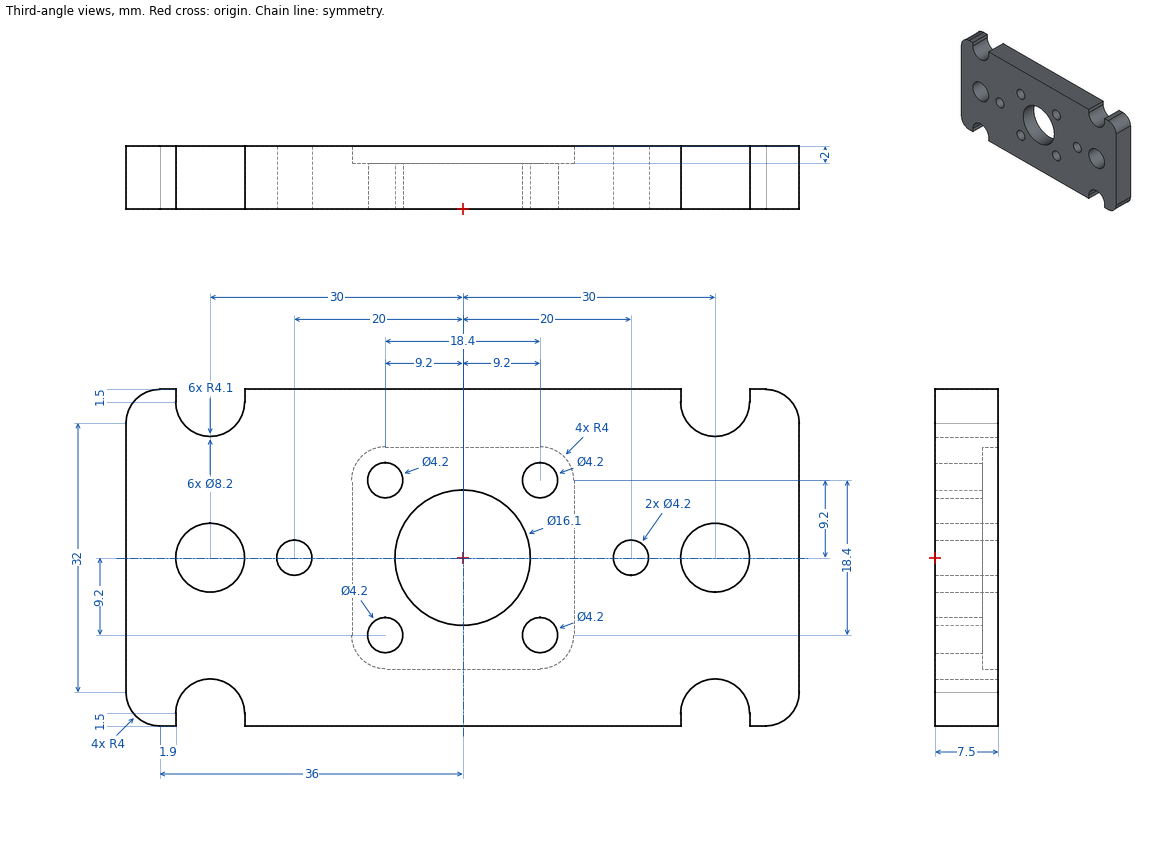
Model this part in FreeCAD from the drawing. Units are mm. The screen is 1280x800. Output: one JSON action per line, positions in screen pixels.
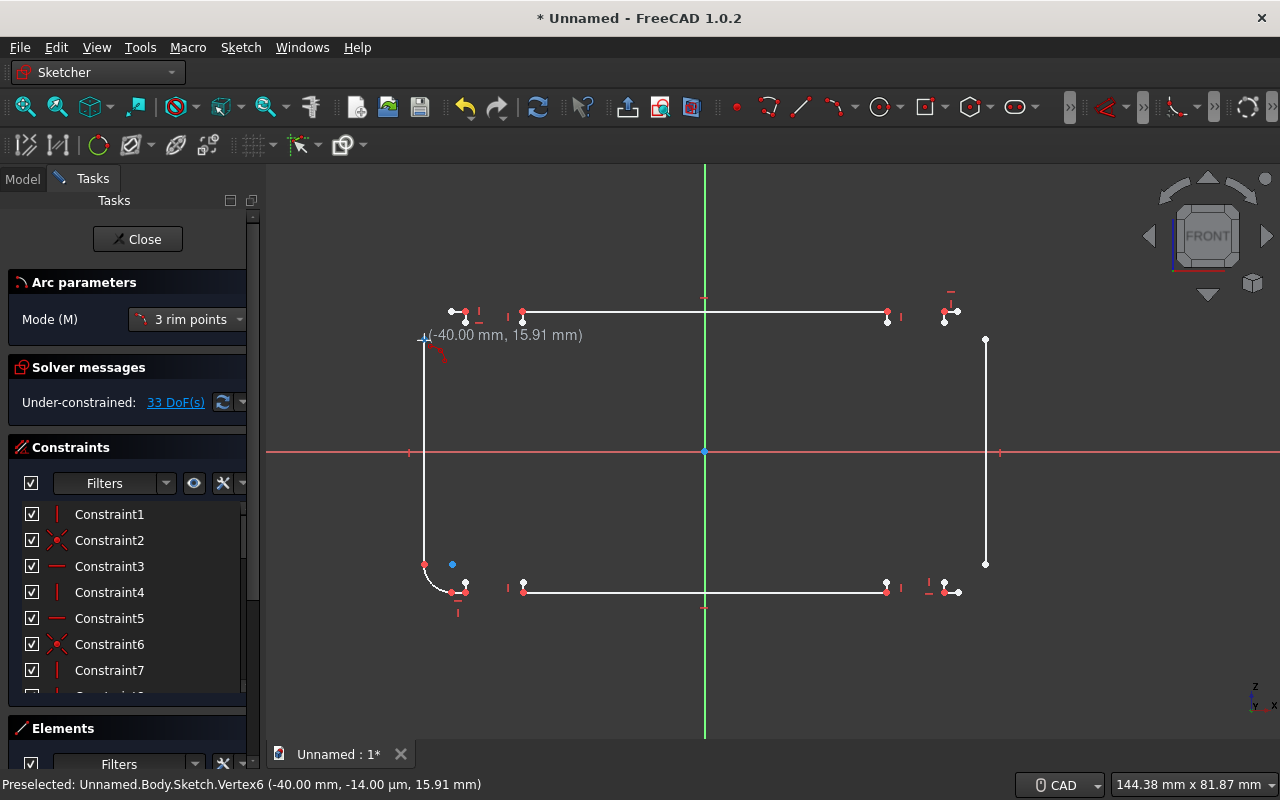
{"action": "scroll", "coordinate": [452, 311], "scroll_direction": "up", "scroll_amount": 5}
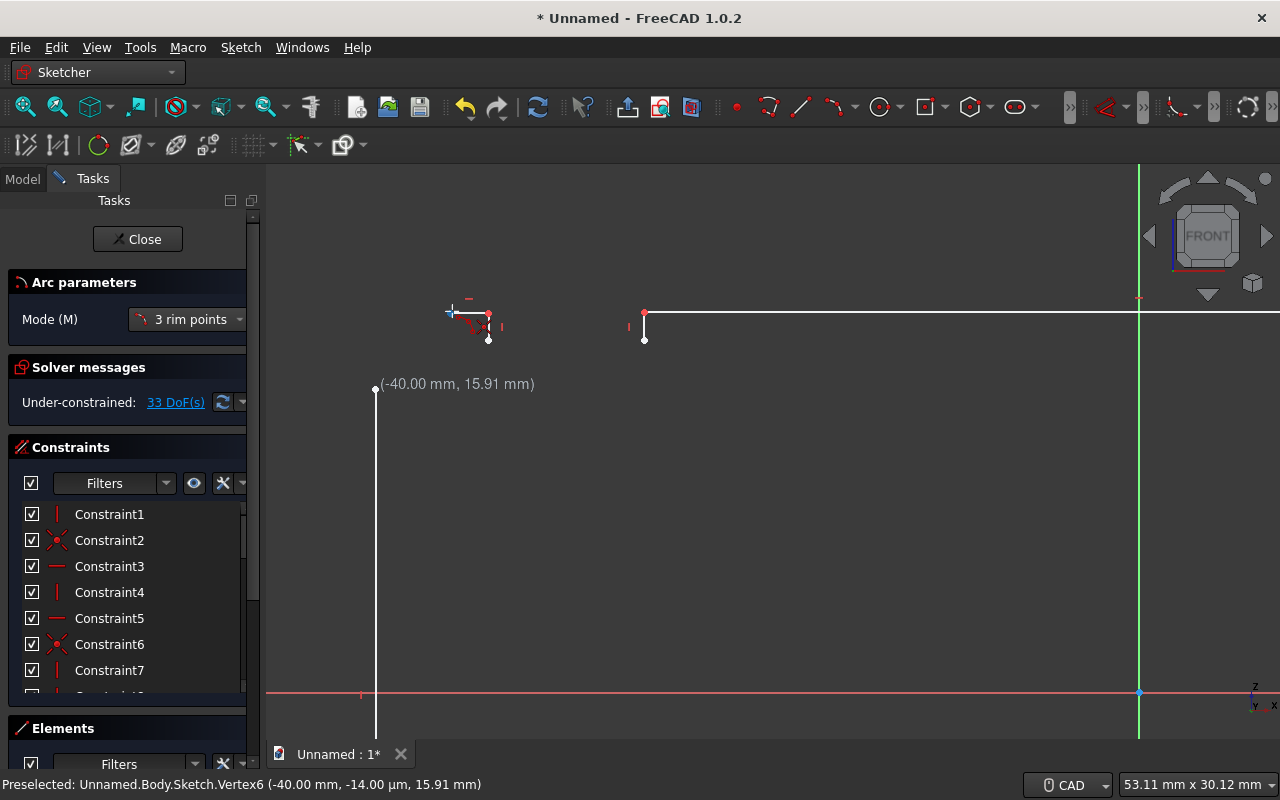
{"action": "left_click", "coordinate": [451, 313]}
{"action": "left_click", "coordinate": [398, 333]}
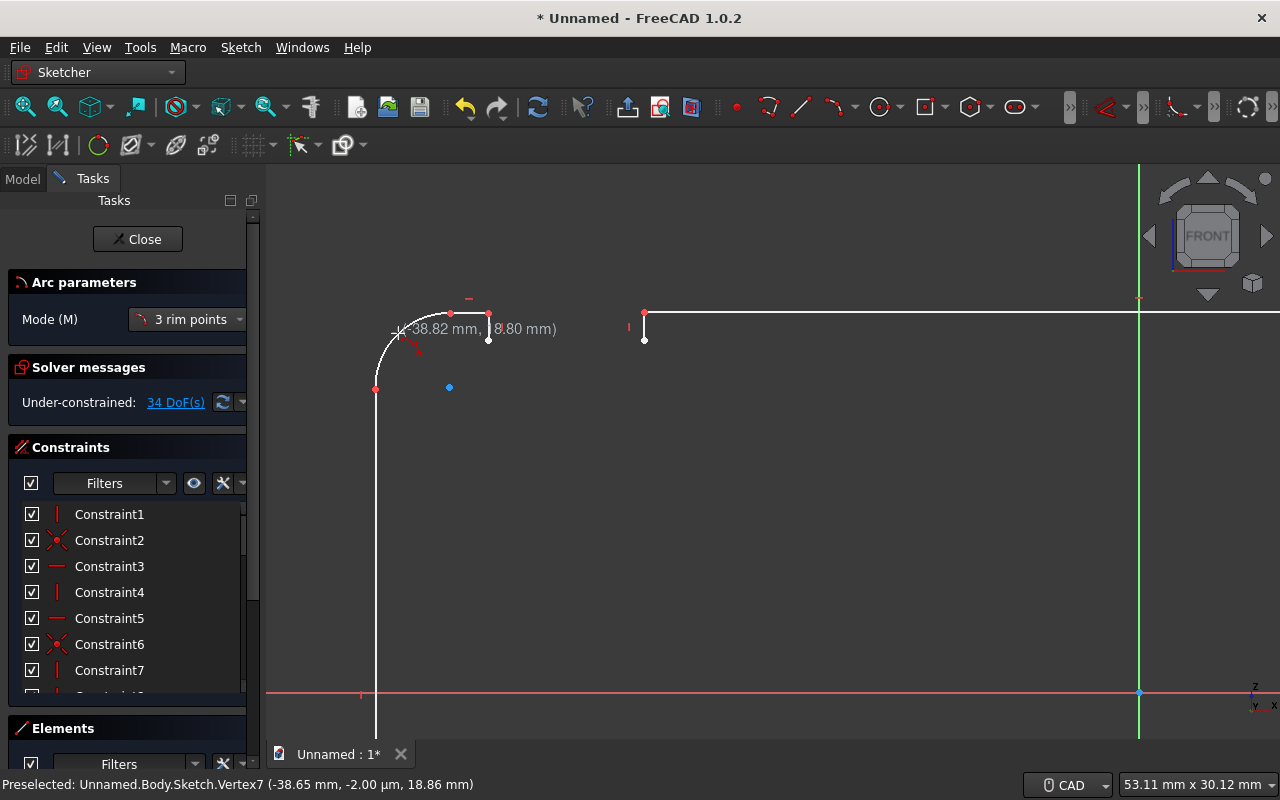
{"action": "left_click", "coordinate": [489, 341]}
{"action": "left_click", "coordinate": [644, 341]}
{"action": "left_click", "coordinate": [566, 418]}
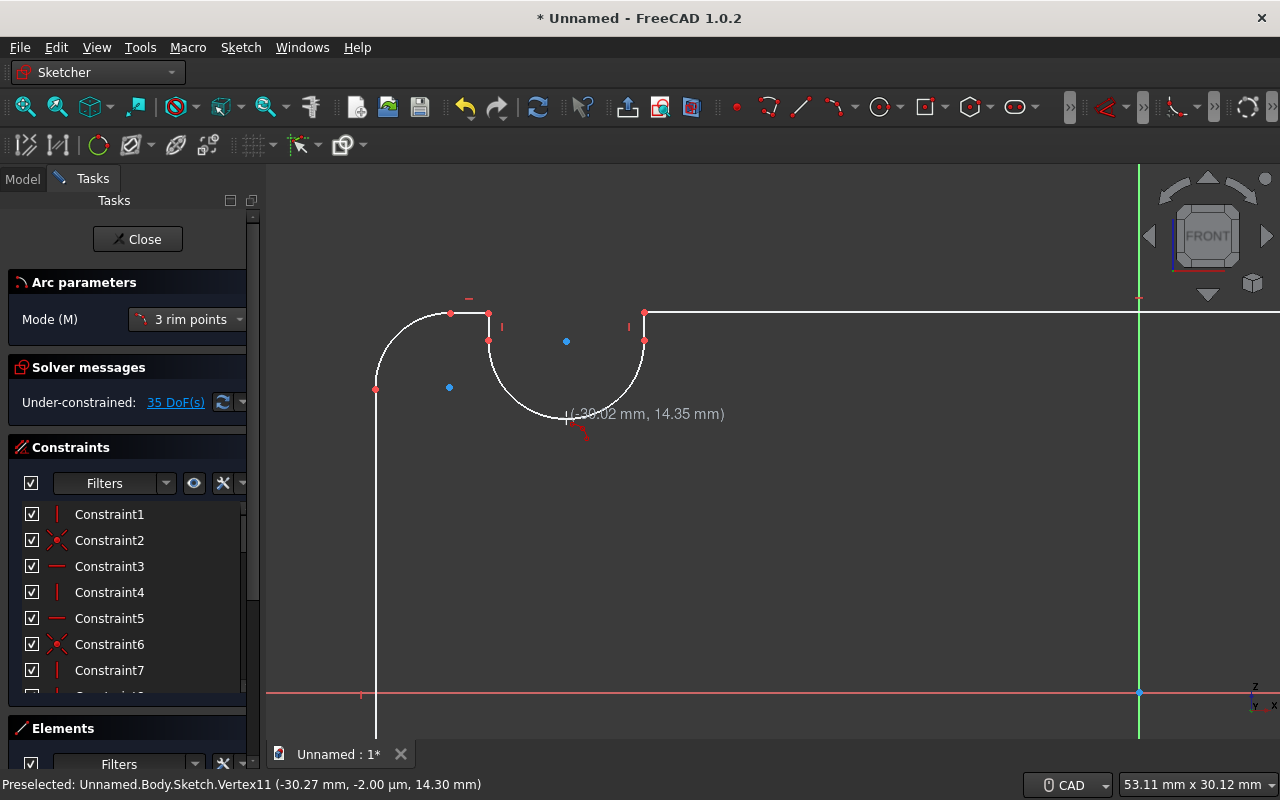
{"action": "scroll", "coordinate": [452, 311], "scroll_direction": "down", "scroll_amount": 5}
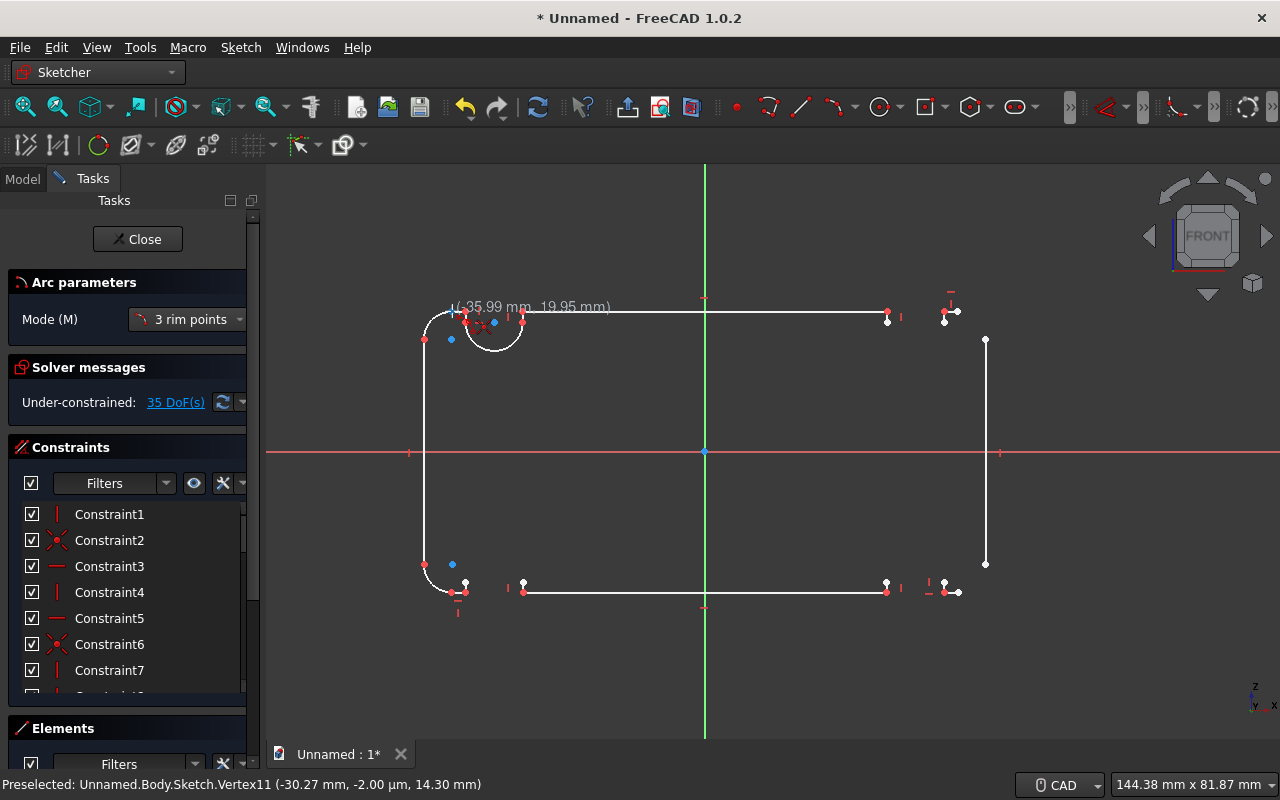
{"action": "scroll", "coordinate": [887, 322], "scroll_direction": "up", "scroll_amount": 6}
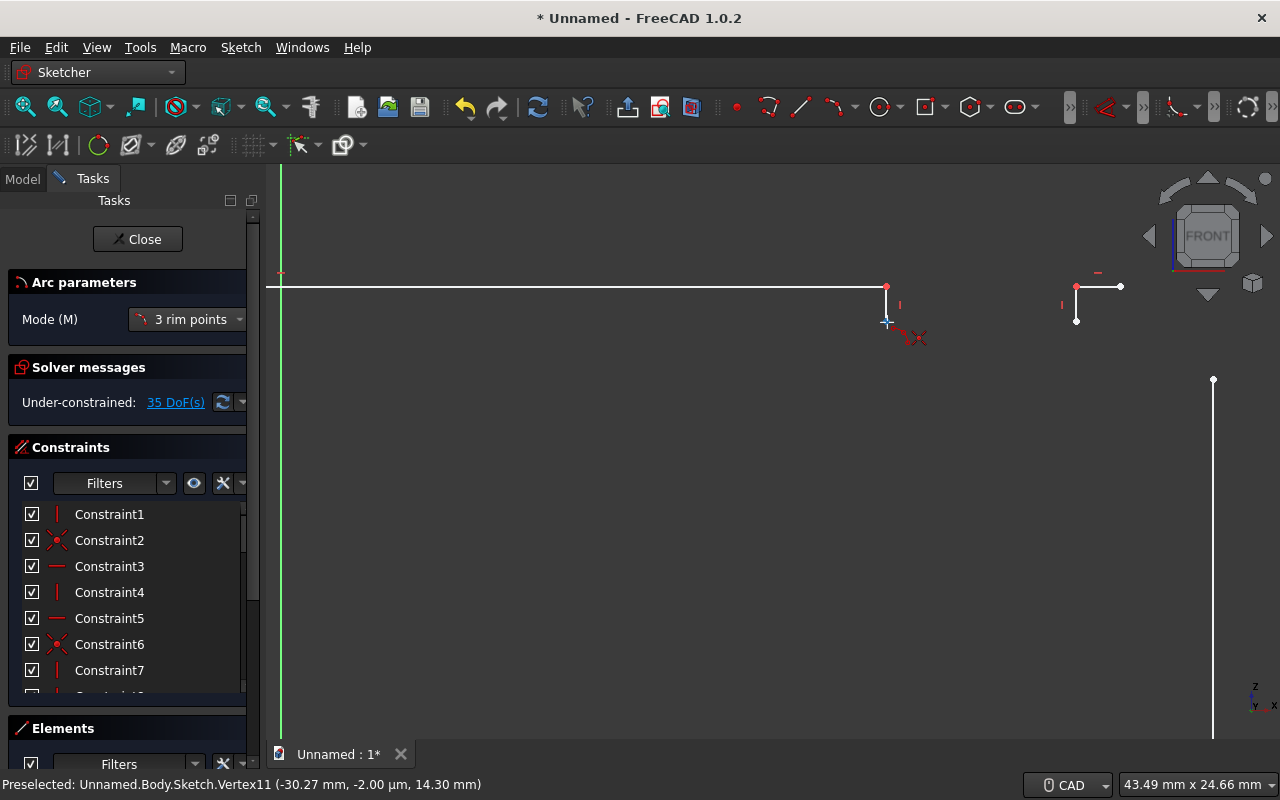
{"action": "left_click", "coordinate": [886, 321]}
{"action": "left_click", "coordinate": [1076, 321]}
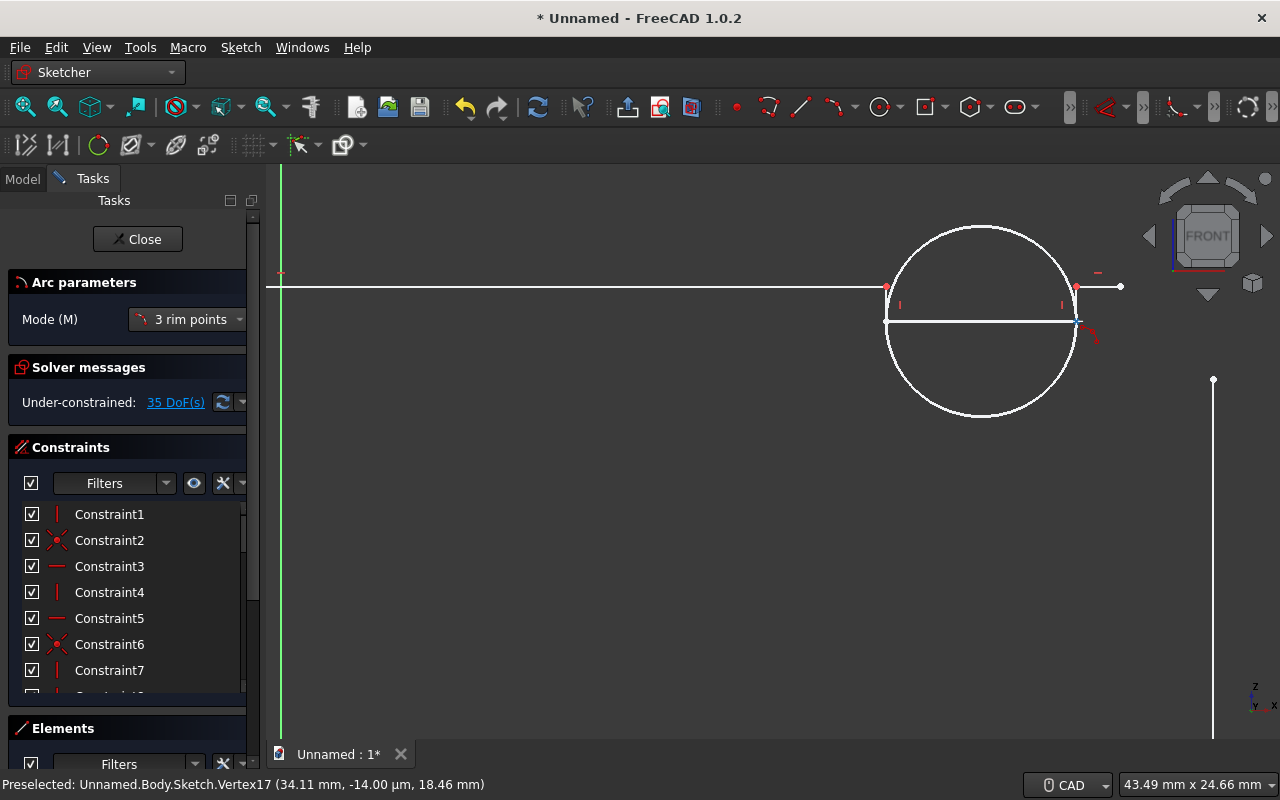
{"action": "scroll", "coordinate": [887, 322], "scroll_direction": "down", "scroll_amount": 6}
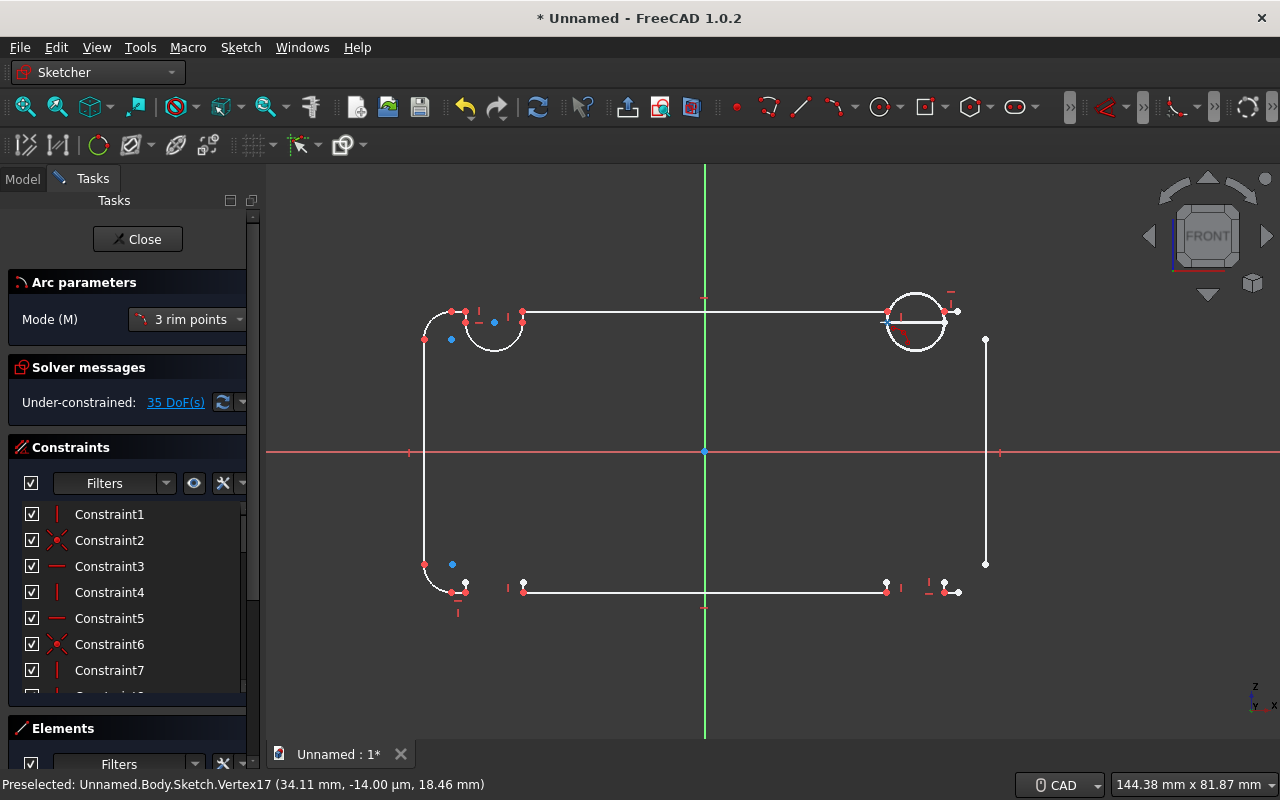
{"action": "left_click", "coordinate": [916, 351]}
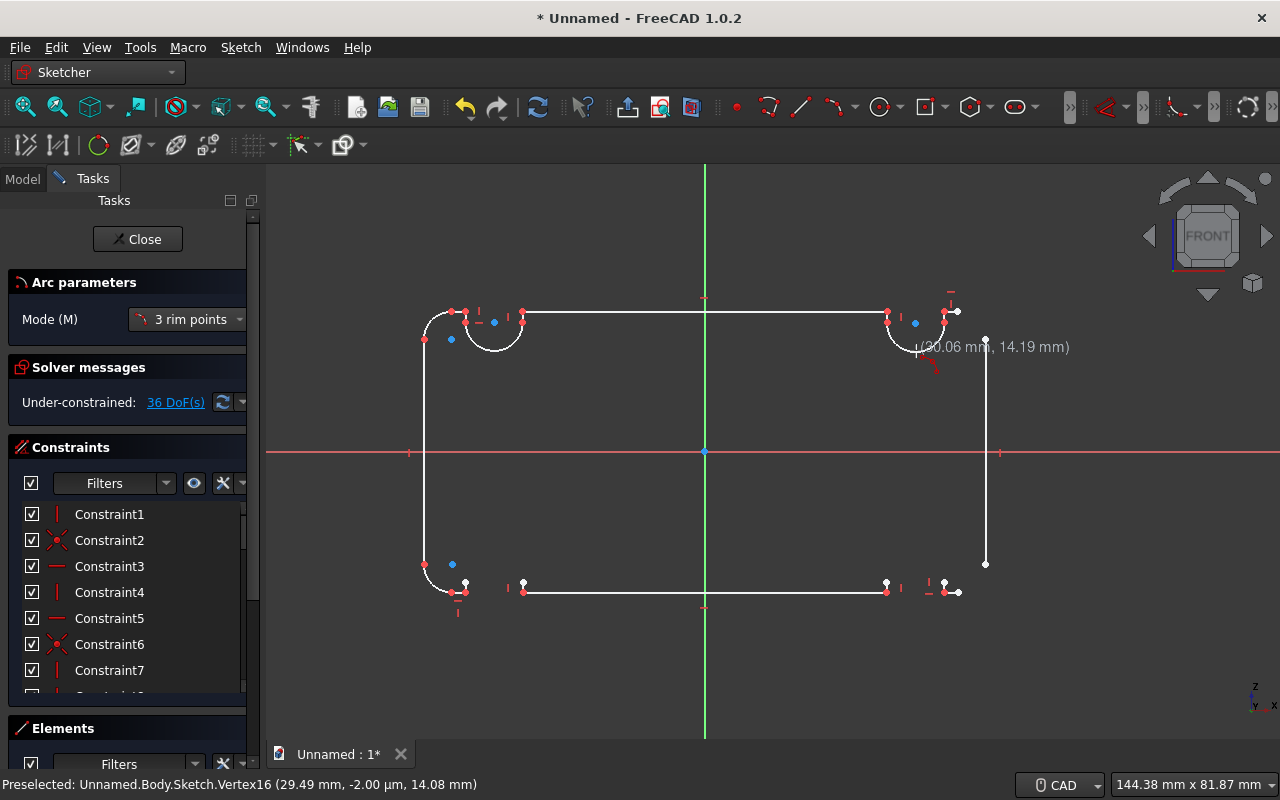
{"action": "scroll", "coordinate": [958, 311], "scroll_direction": "up", "scroll_amount": 5}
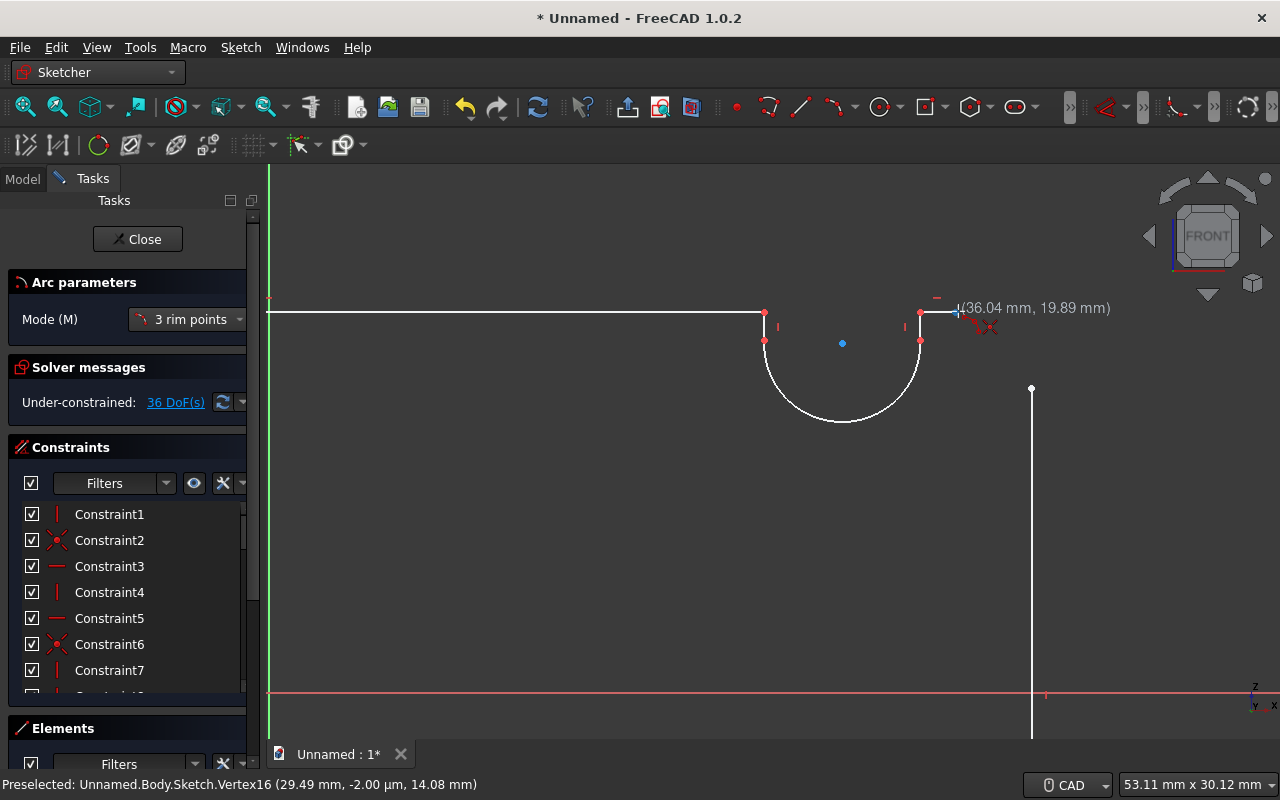
{"action": "left_click", "coordinate": [956, 312]}
{"action": "left_click", "coordinate": [1032, 388]}
{"action": "left_click", "coordinate": [1010, 333]}